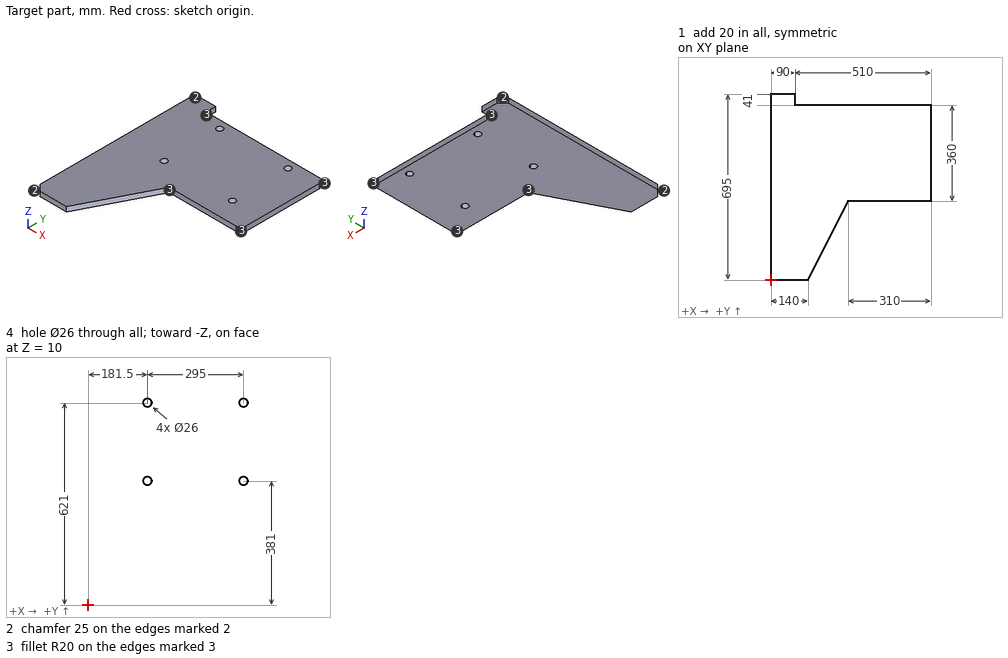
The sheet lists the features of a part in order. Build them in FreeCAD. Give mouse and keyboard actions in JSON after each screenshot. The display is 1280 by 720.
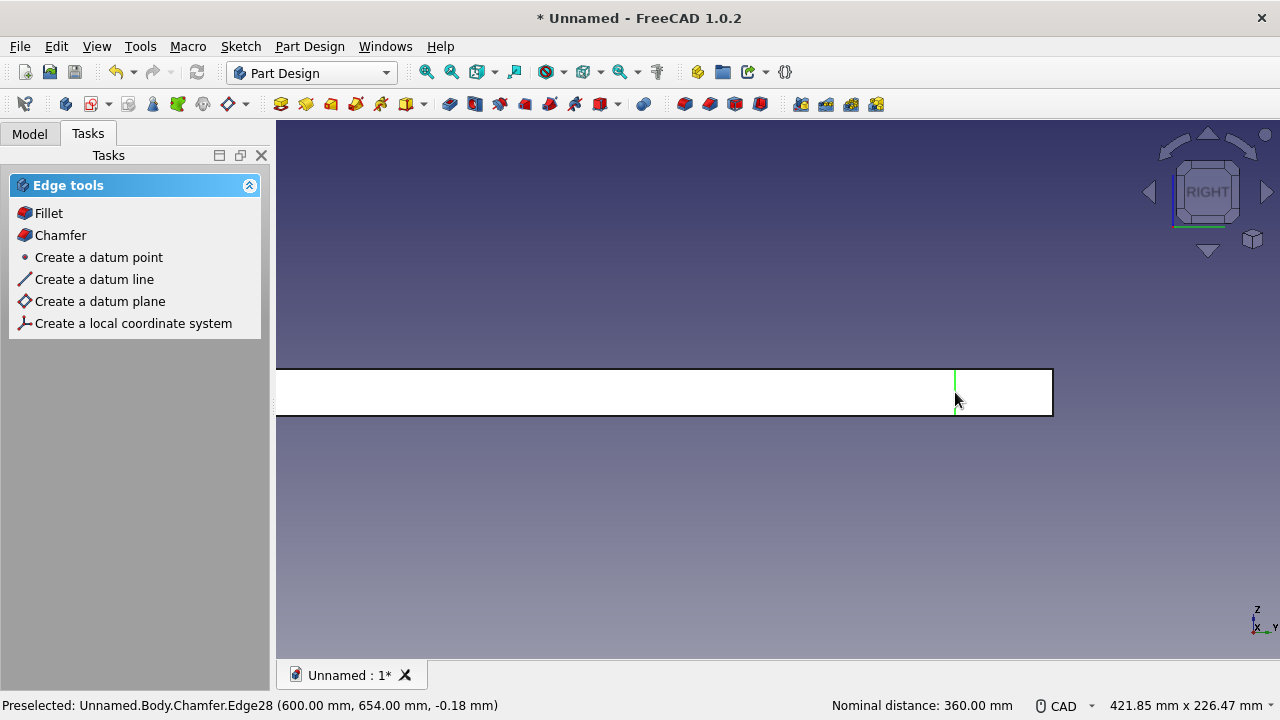
{"action": "left_click", "coordinate": [427, 72]}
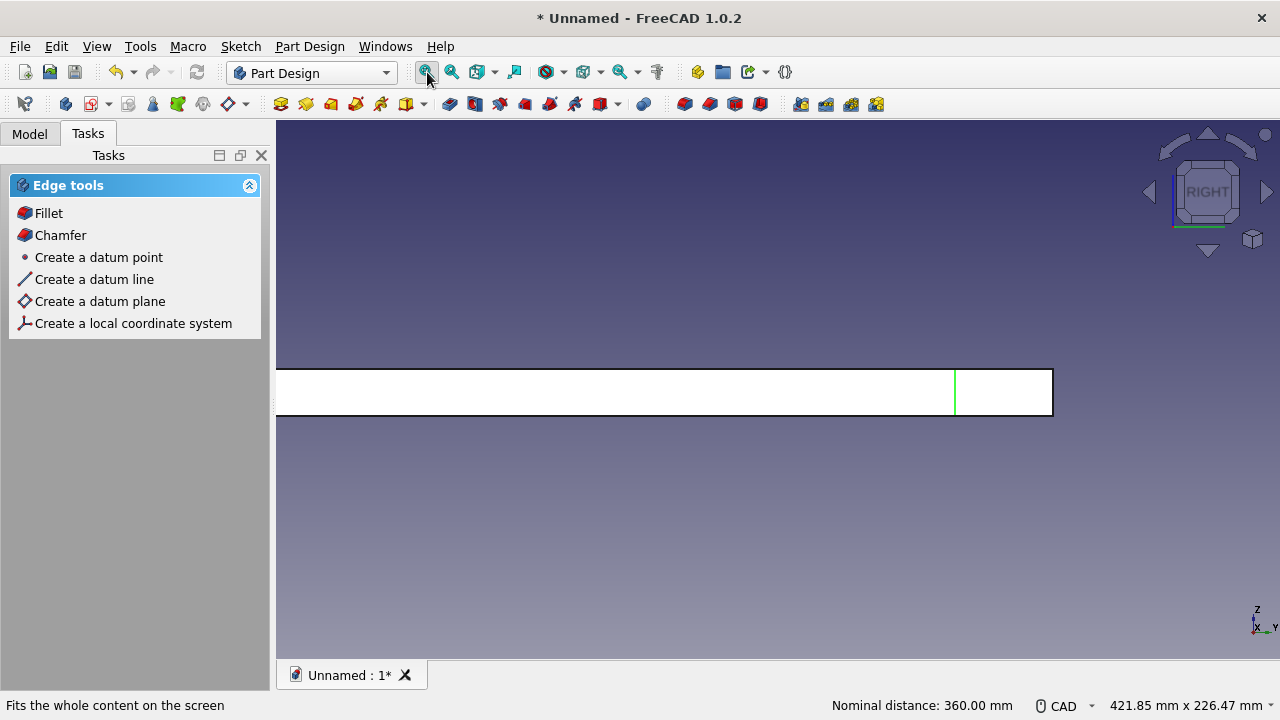
{"action": "key", "text": "5"}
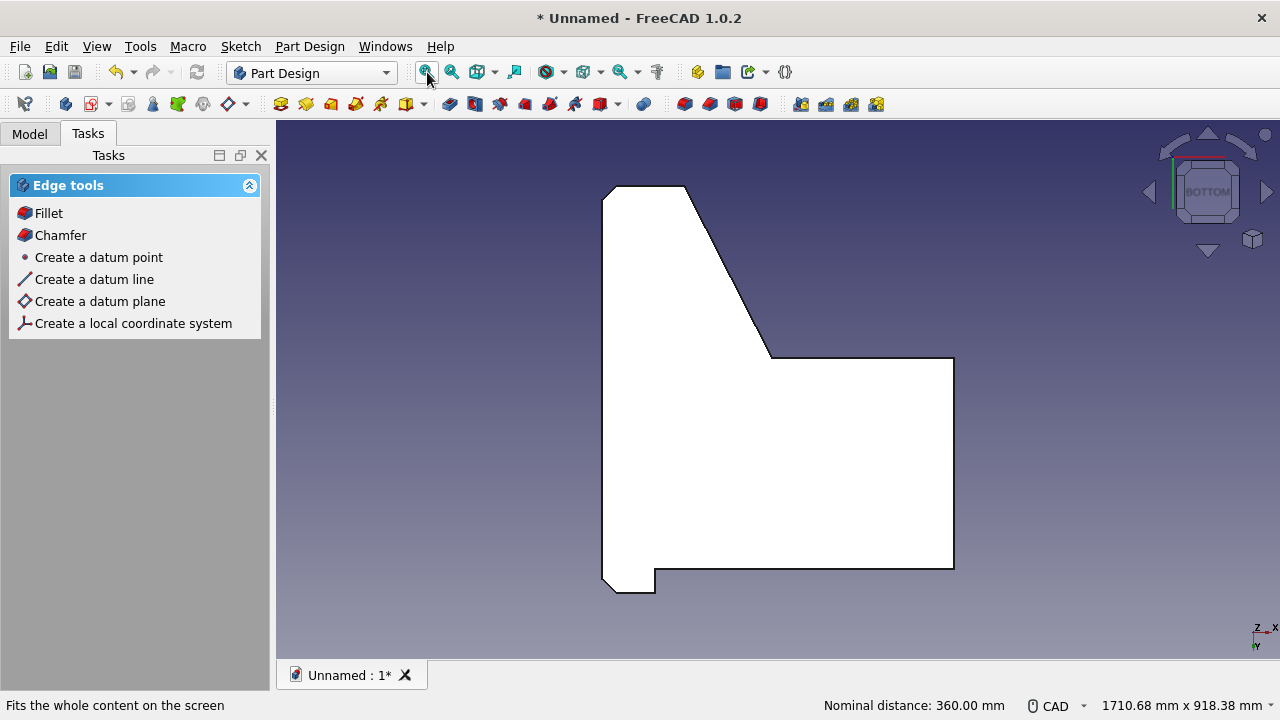
{"action": "scroll", "coordinate": [655, 568], "scroll_direction": "up", "scroll_amount": 7}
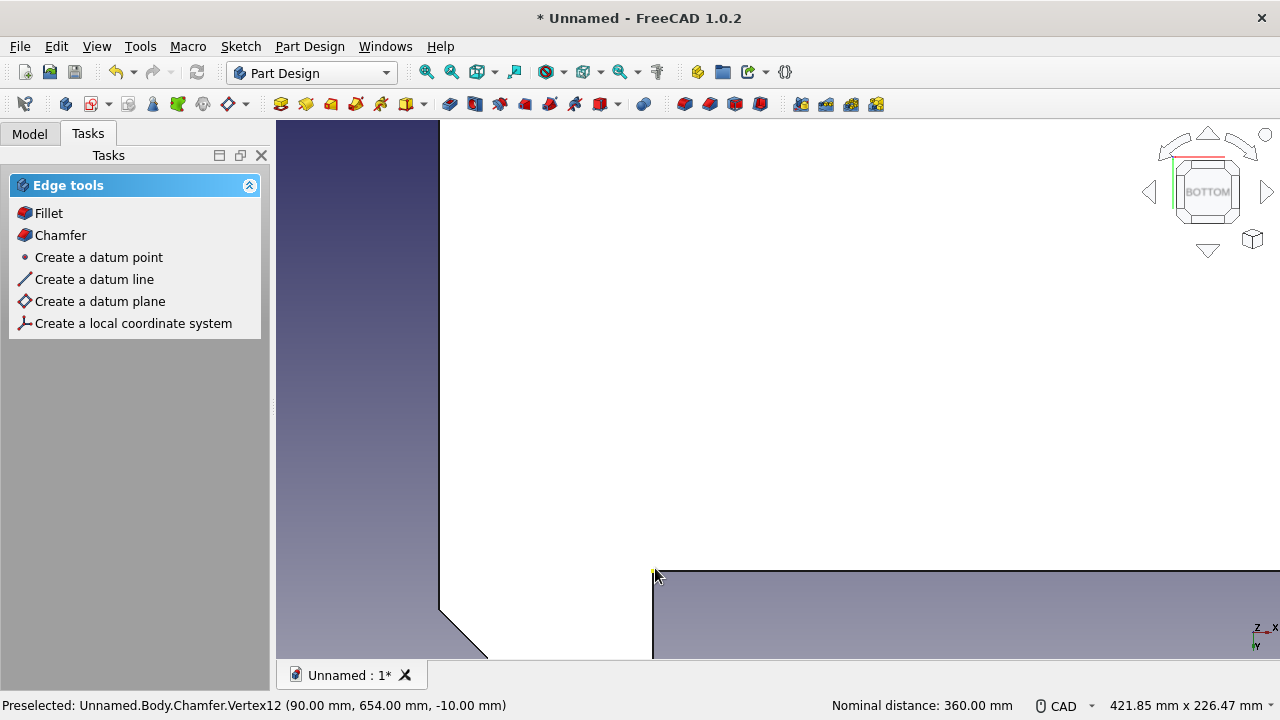
{"action": "left_click", "coordinate": [427, 72]}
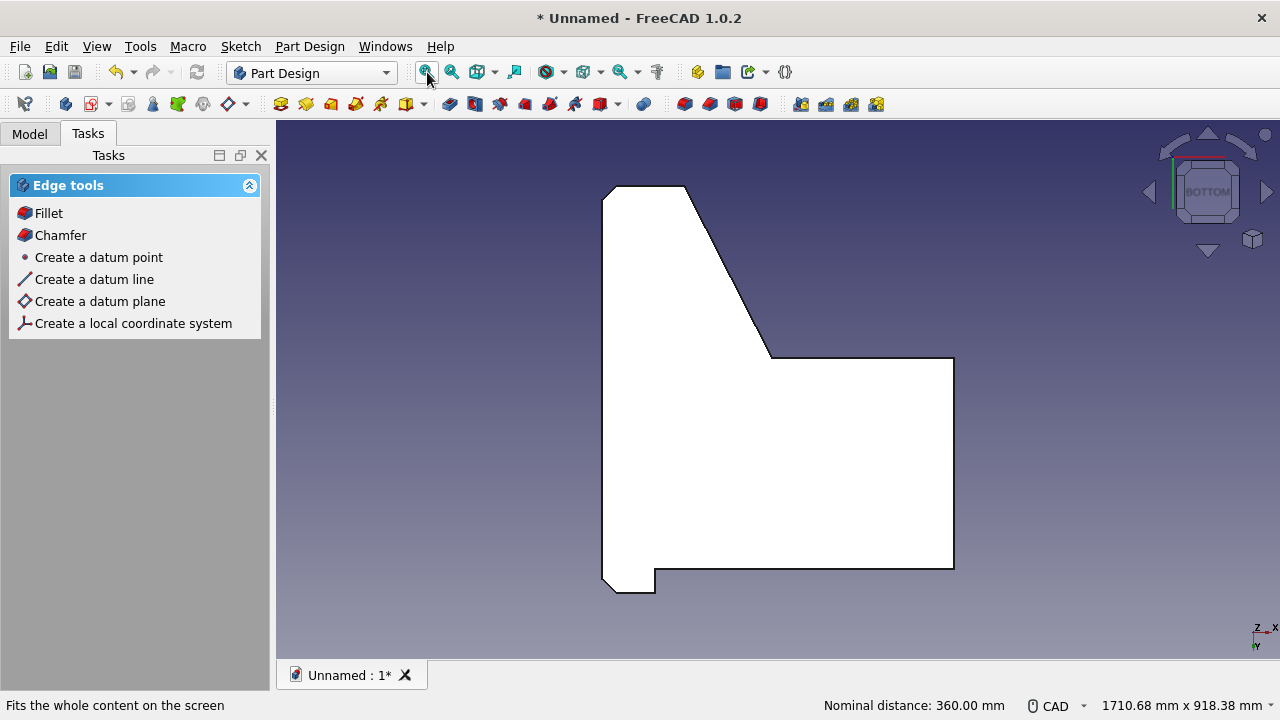
{"action": "key", "text": "4"}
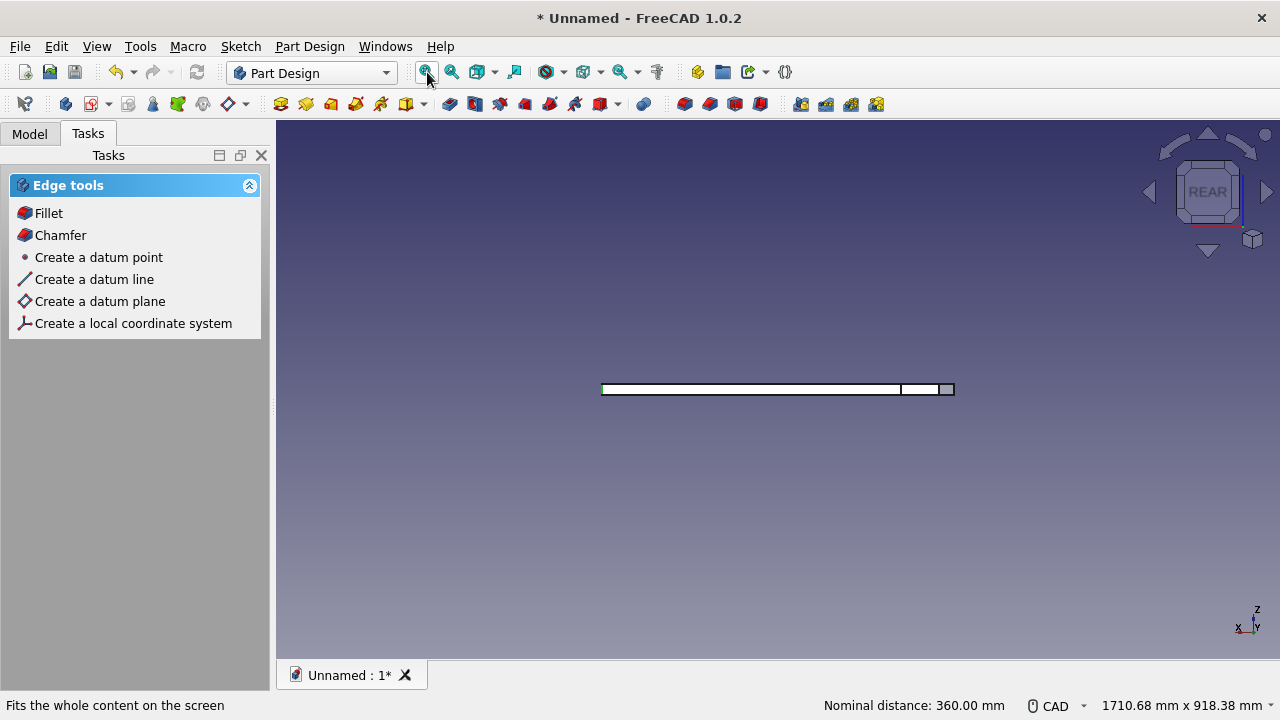
{"action": "left_click", "coordinate": [427, 72]}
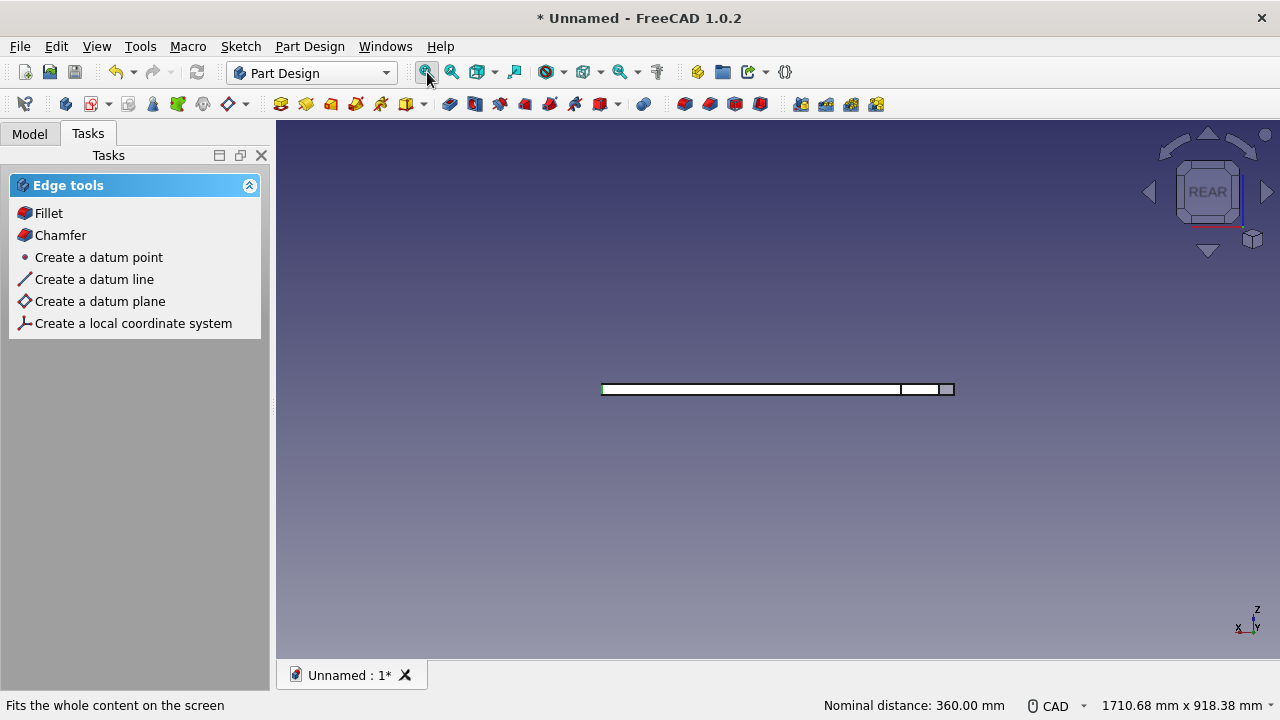
{"action": "scroll", "coordinate": [901, 389], "scroll_direction": "up", "scroll_amount": 7}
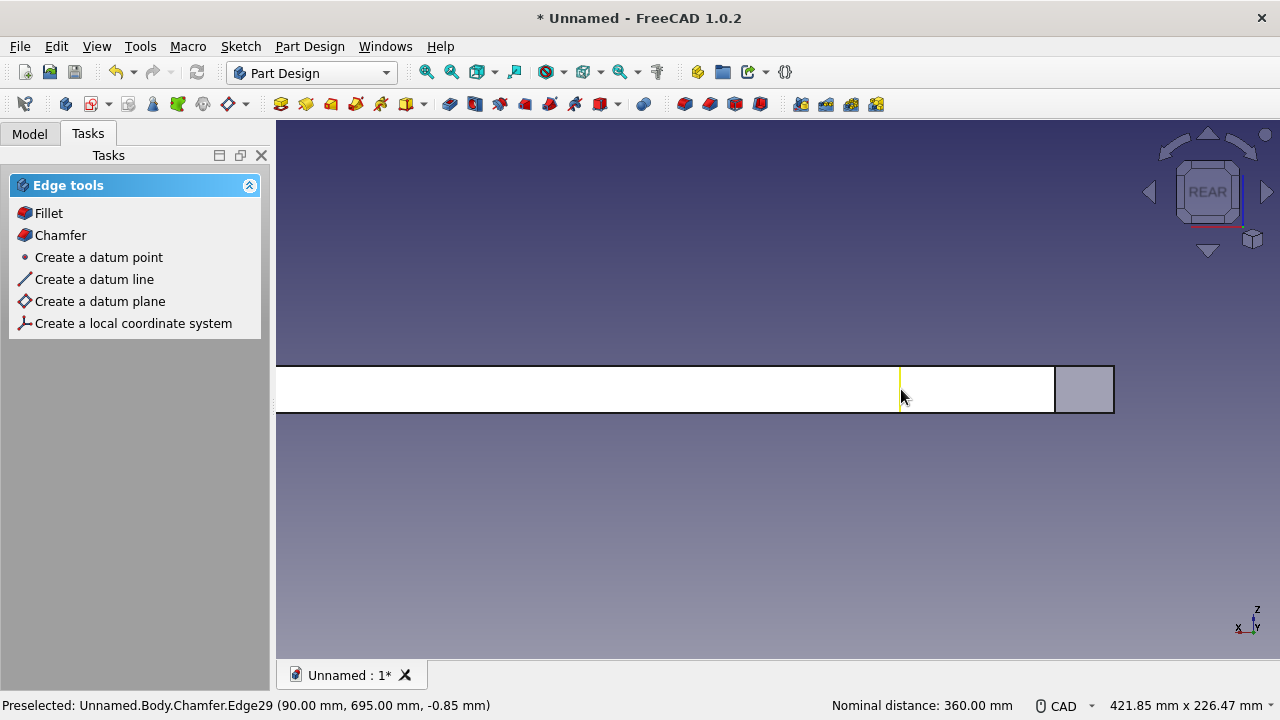
{"action": "left_click", "coordinate": [427, 72]}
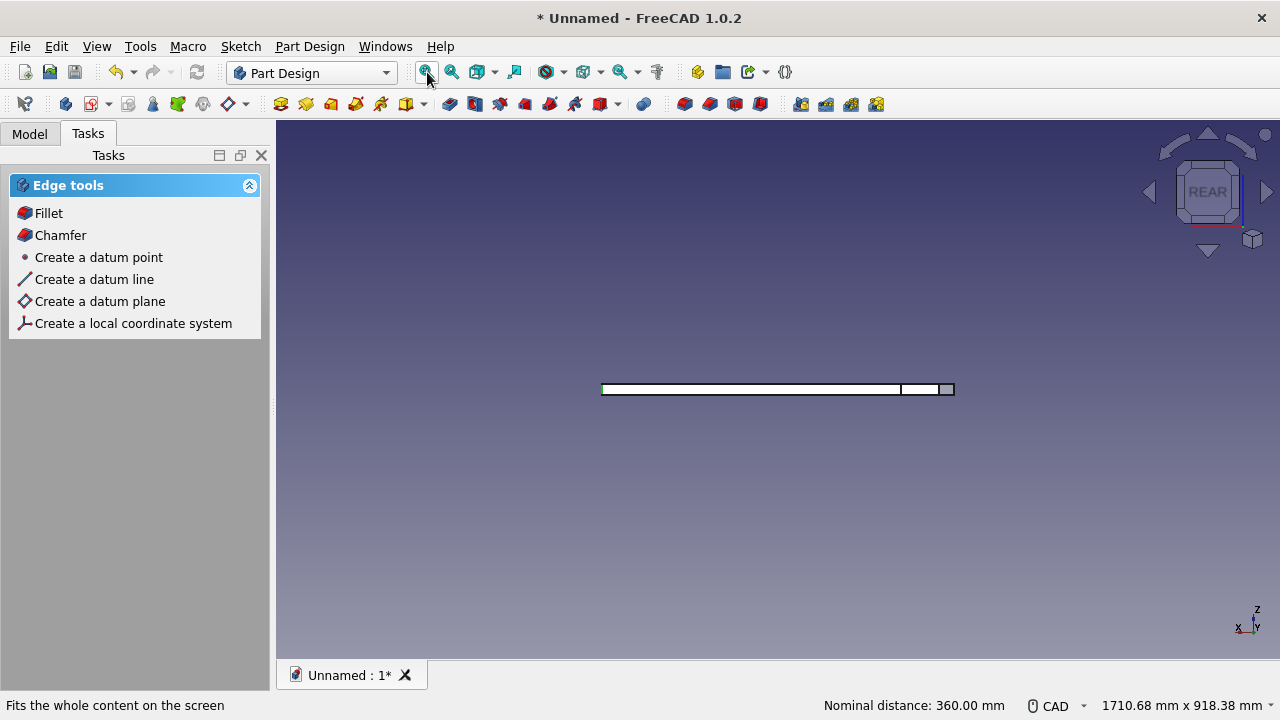
{"action": "key", "text": "6"}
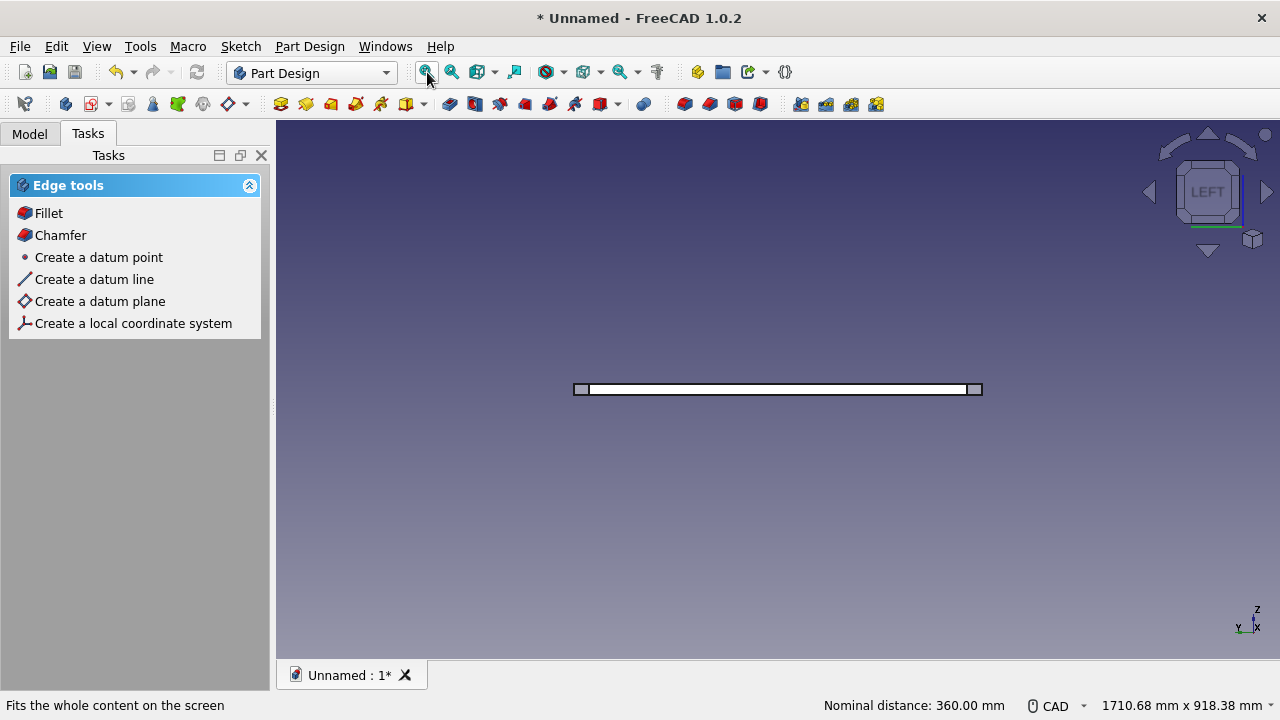
{"action": "left_click", "coordinate": [427, 72]}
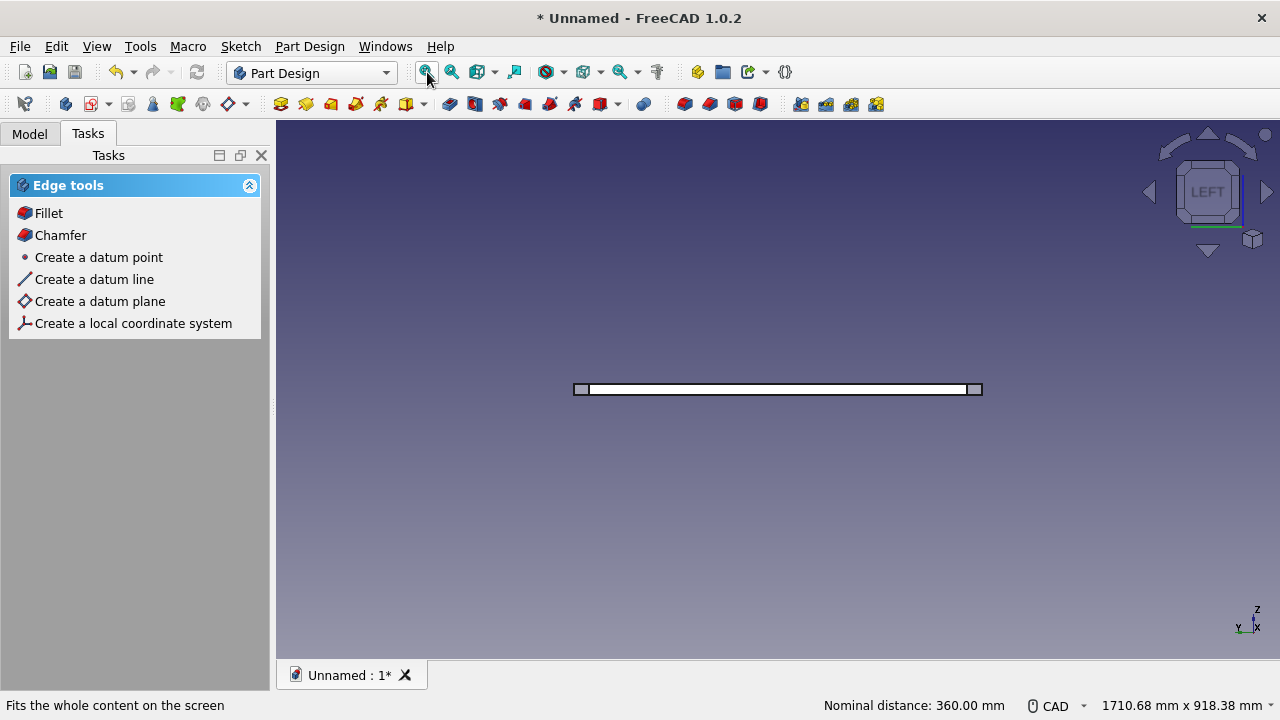
{"action": "scroll", "coordinate": [598, 388], "scroll_direction": "up", "scroll_amount": 7}